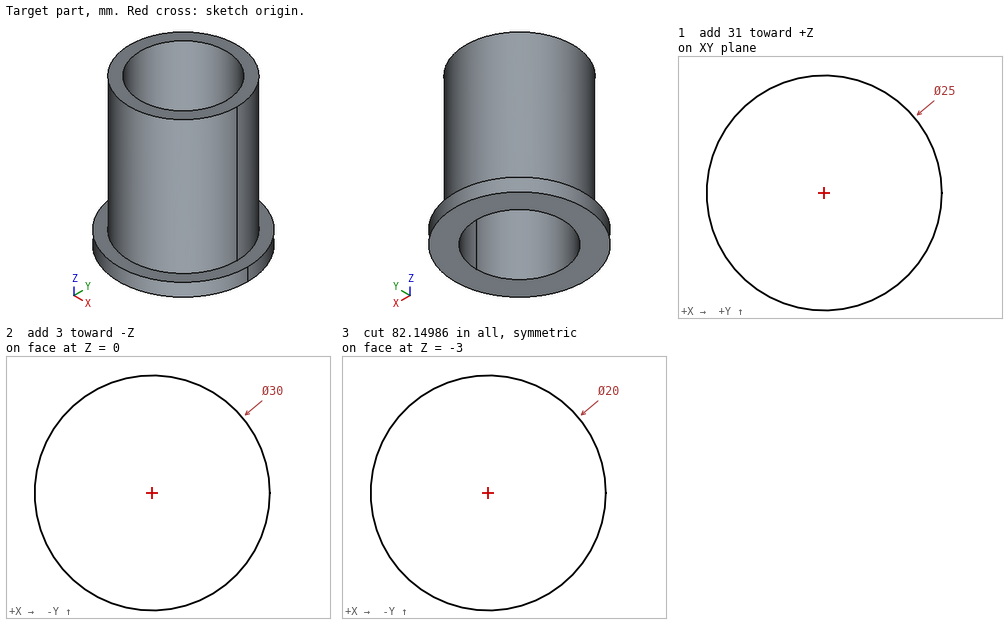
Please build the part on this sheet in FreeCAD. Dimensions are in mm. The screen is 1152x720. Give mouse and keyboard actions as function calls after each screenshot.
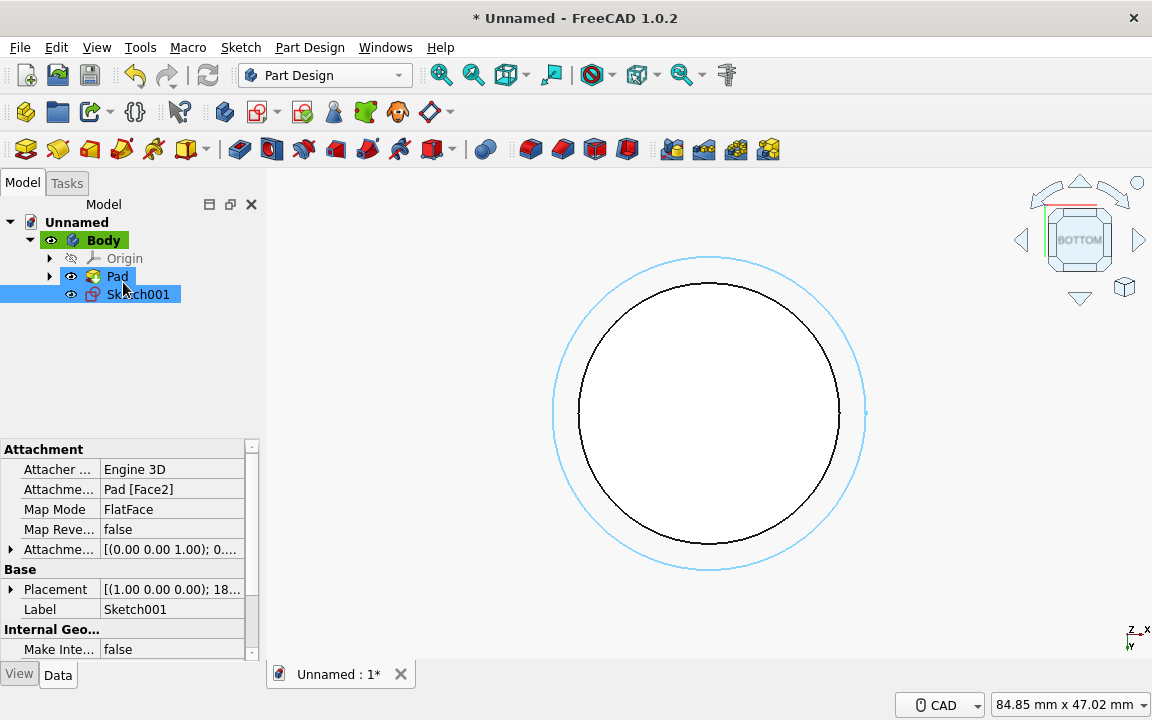
click(26, 150)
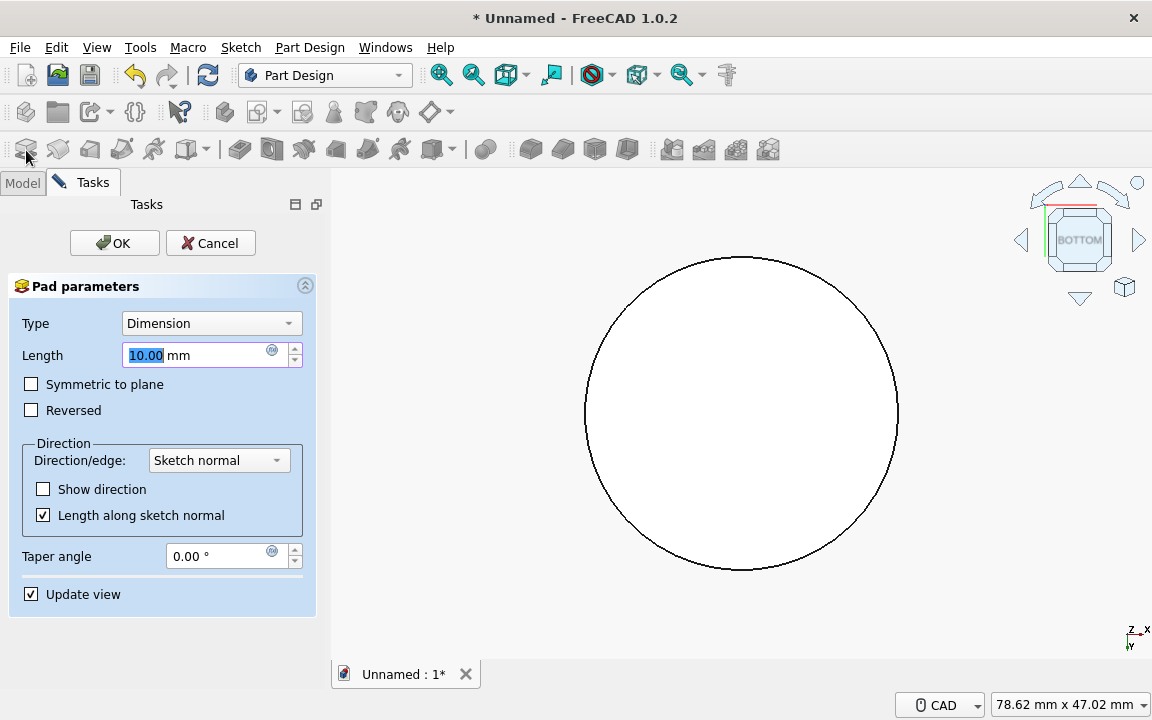
text(3)
key(Tab)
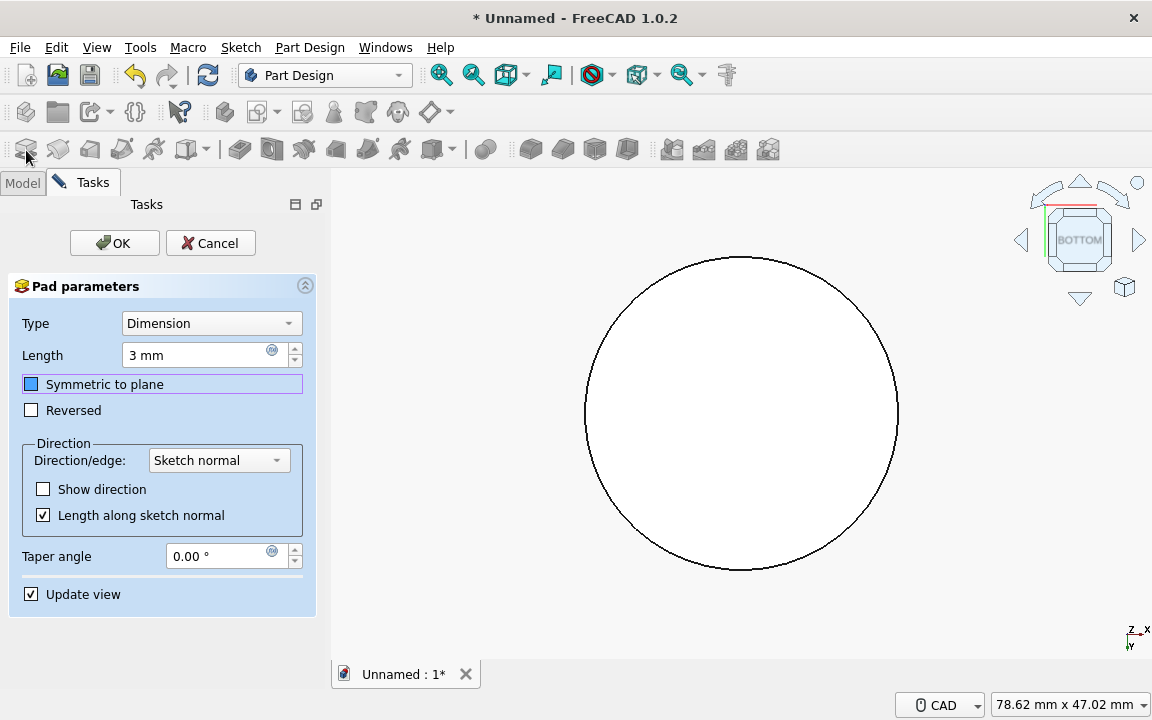
click(115, 243)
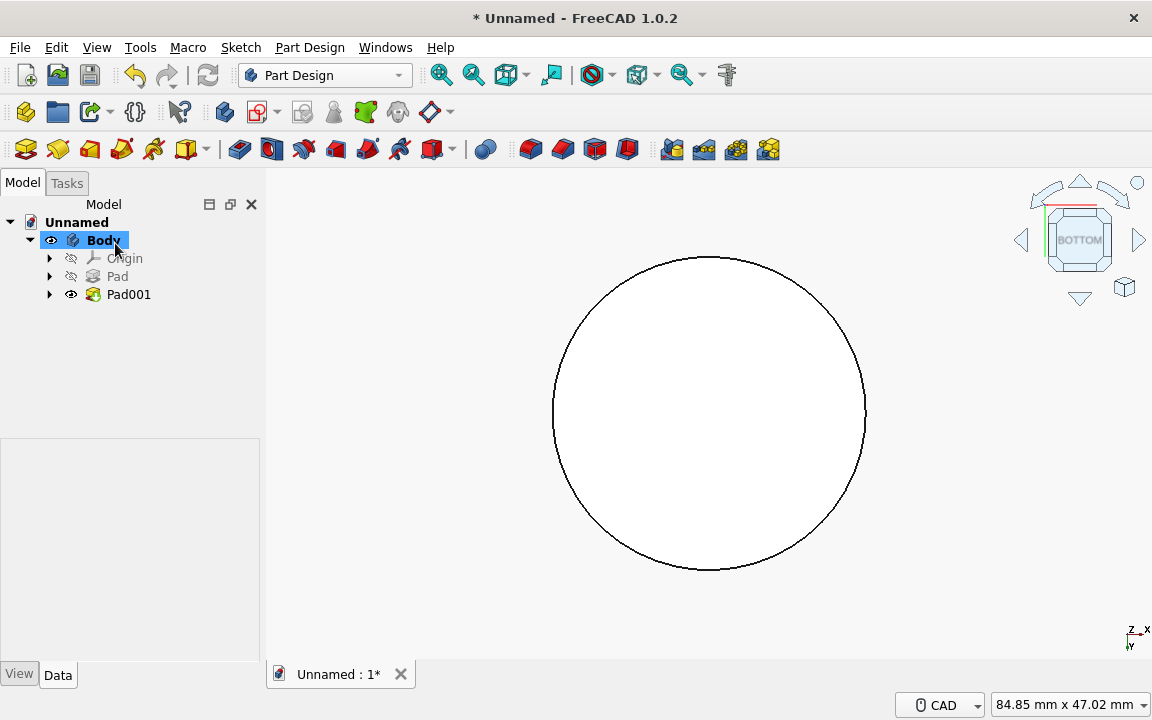
click(709, 413)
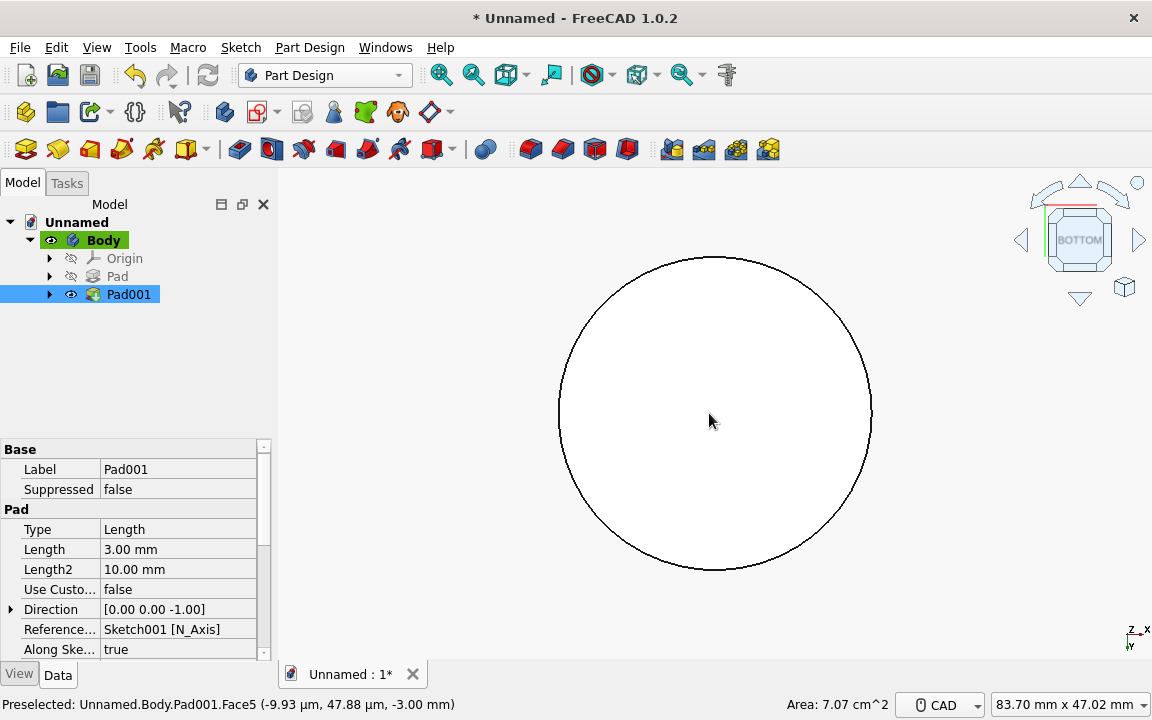
click(258, 112)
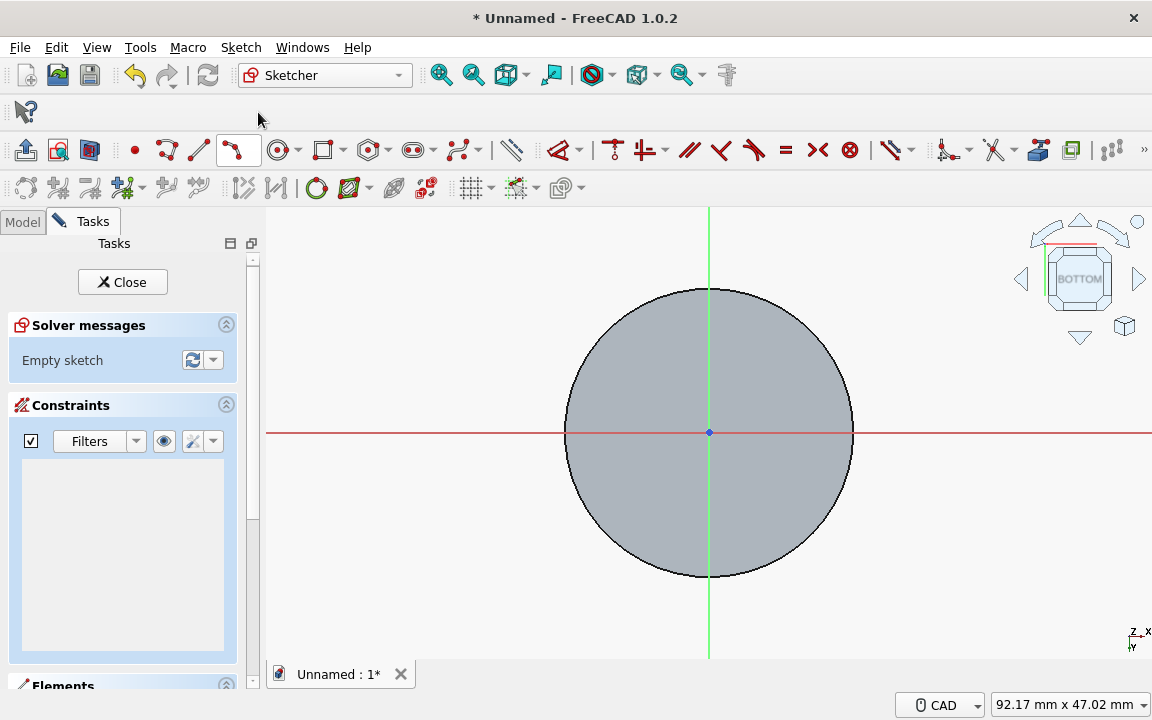
scroll(849, 433, up, 2)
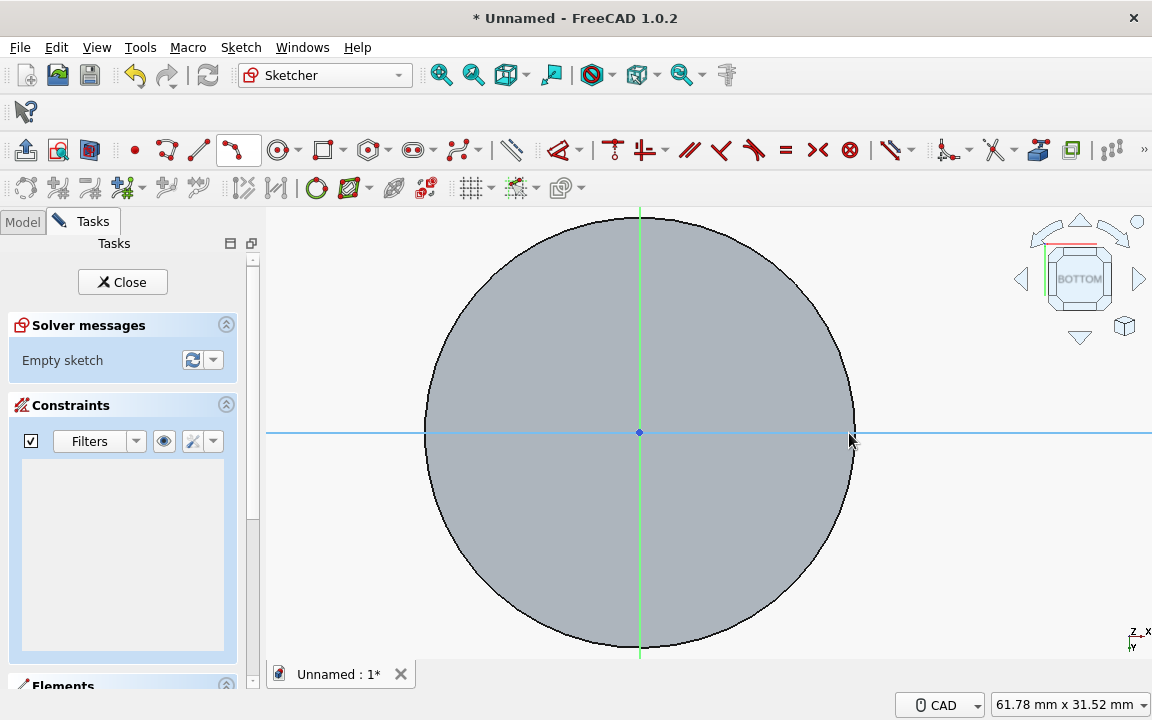
click(278, 150)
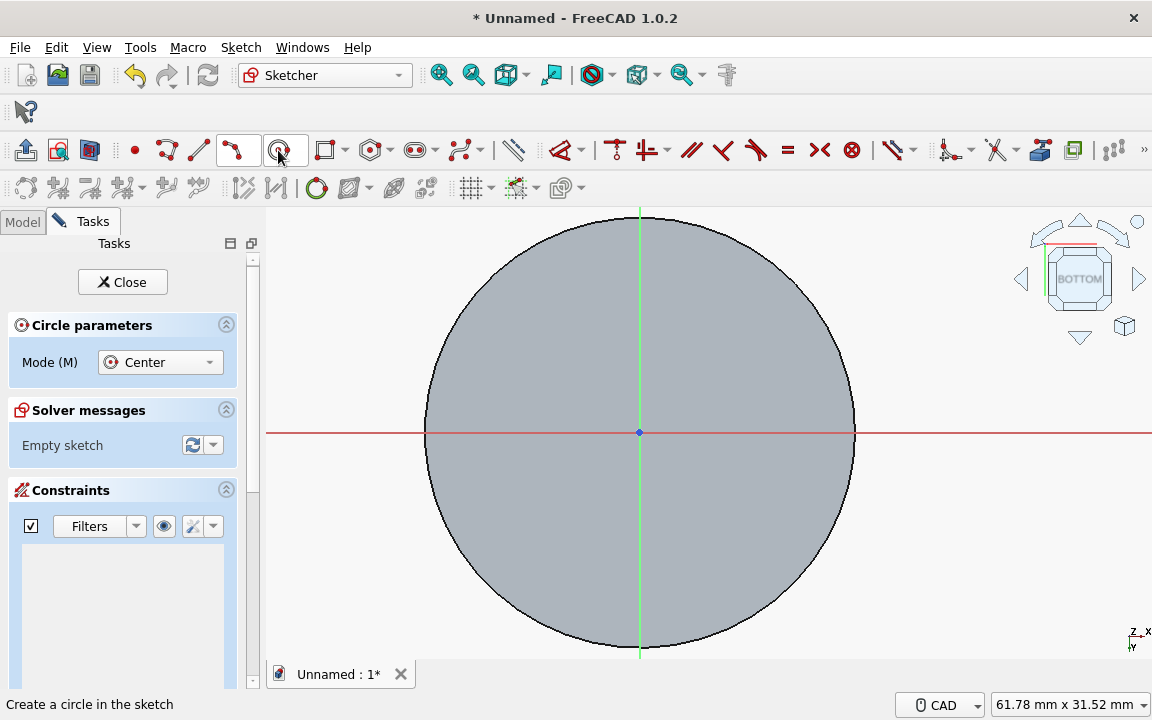
click(640, 433)
click(741, 331)
key(Escape)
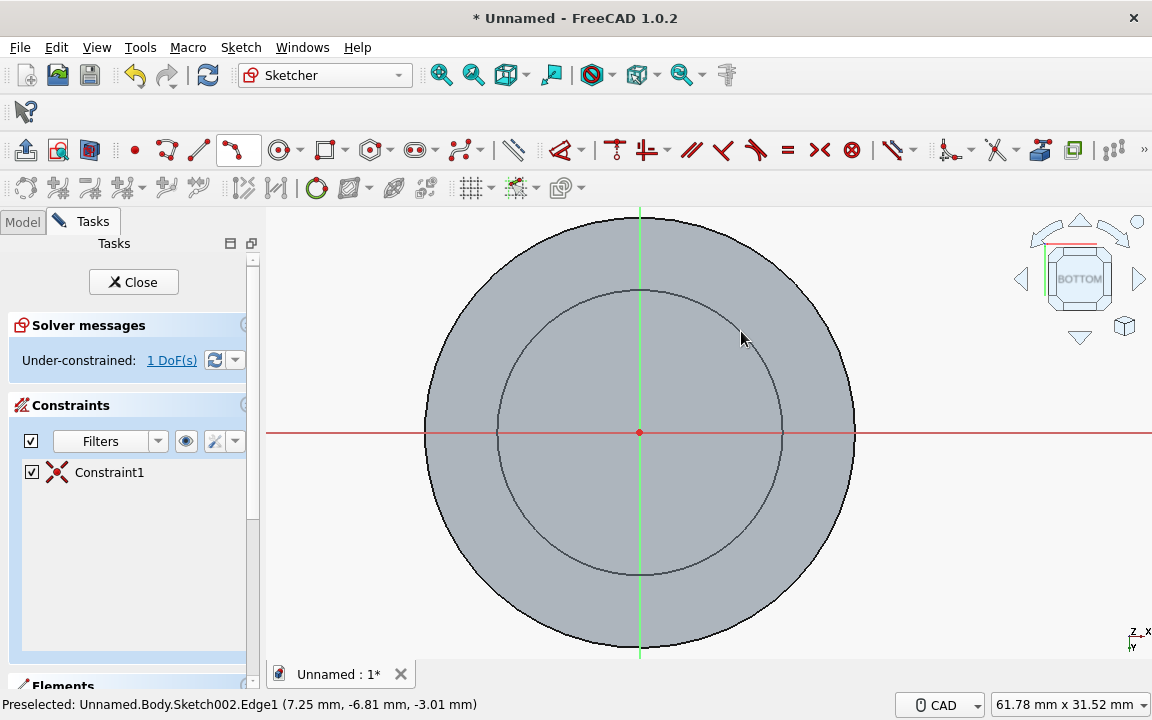
click(560, 150)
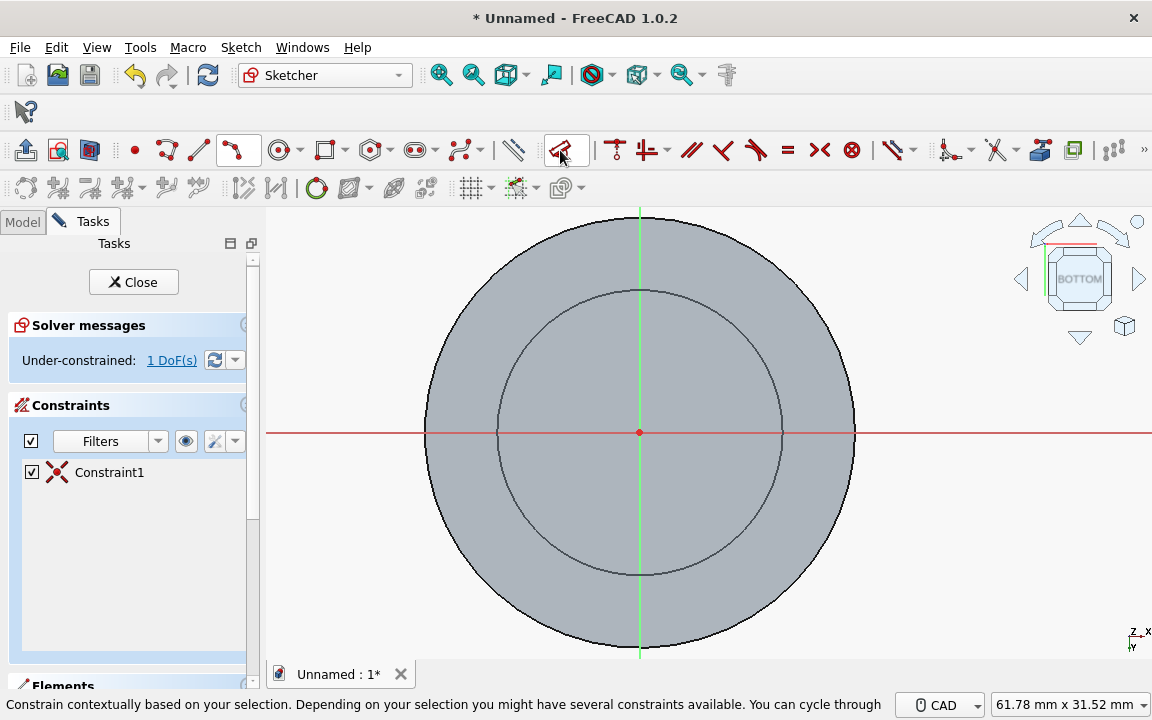
click(741, 332)
click(764, 309)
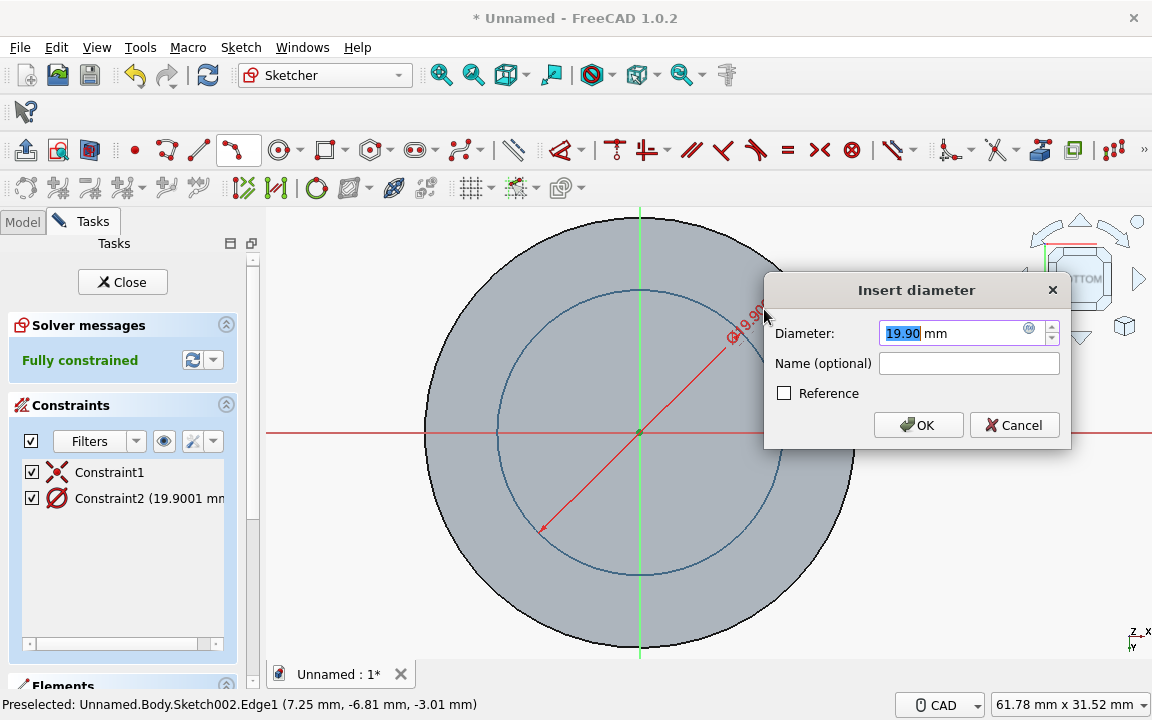
text(20)
key(Return)
key(Escape)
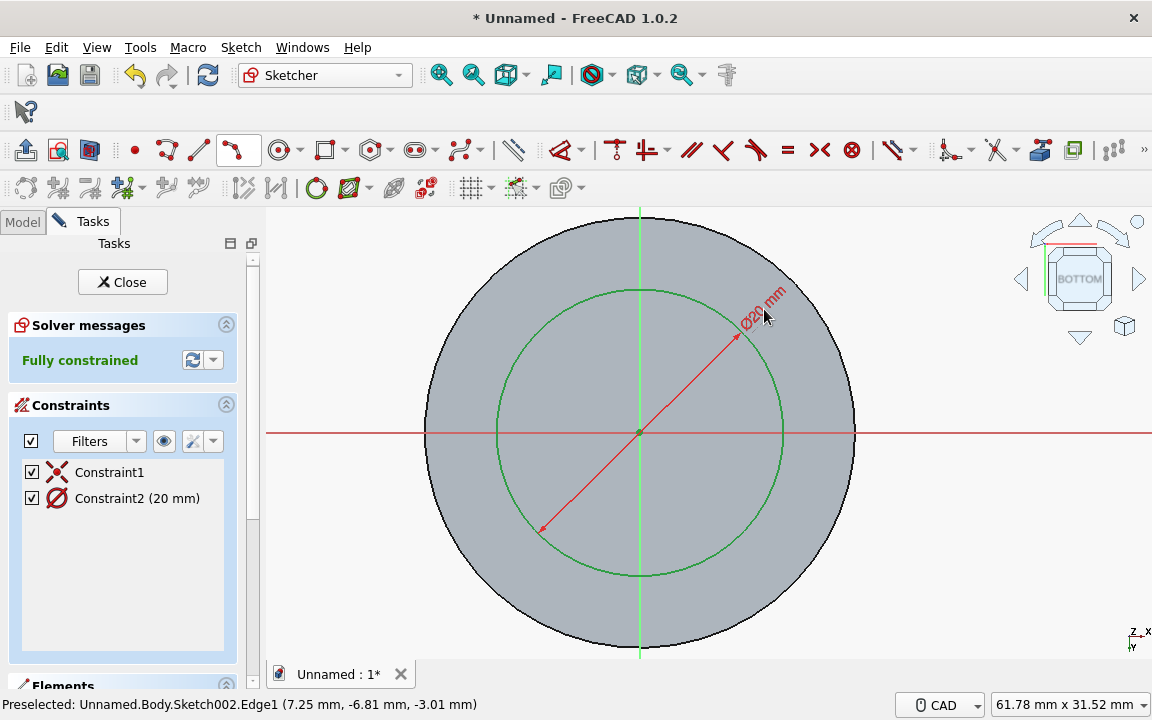
click(123, 282)